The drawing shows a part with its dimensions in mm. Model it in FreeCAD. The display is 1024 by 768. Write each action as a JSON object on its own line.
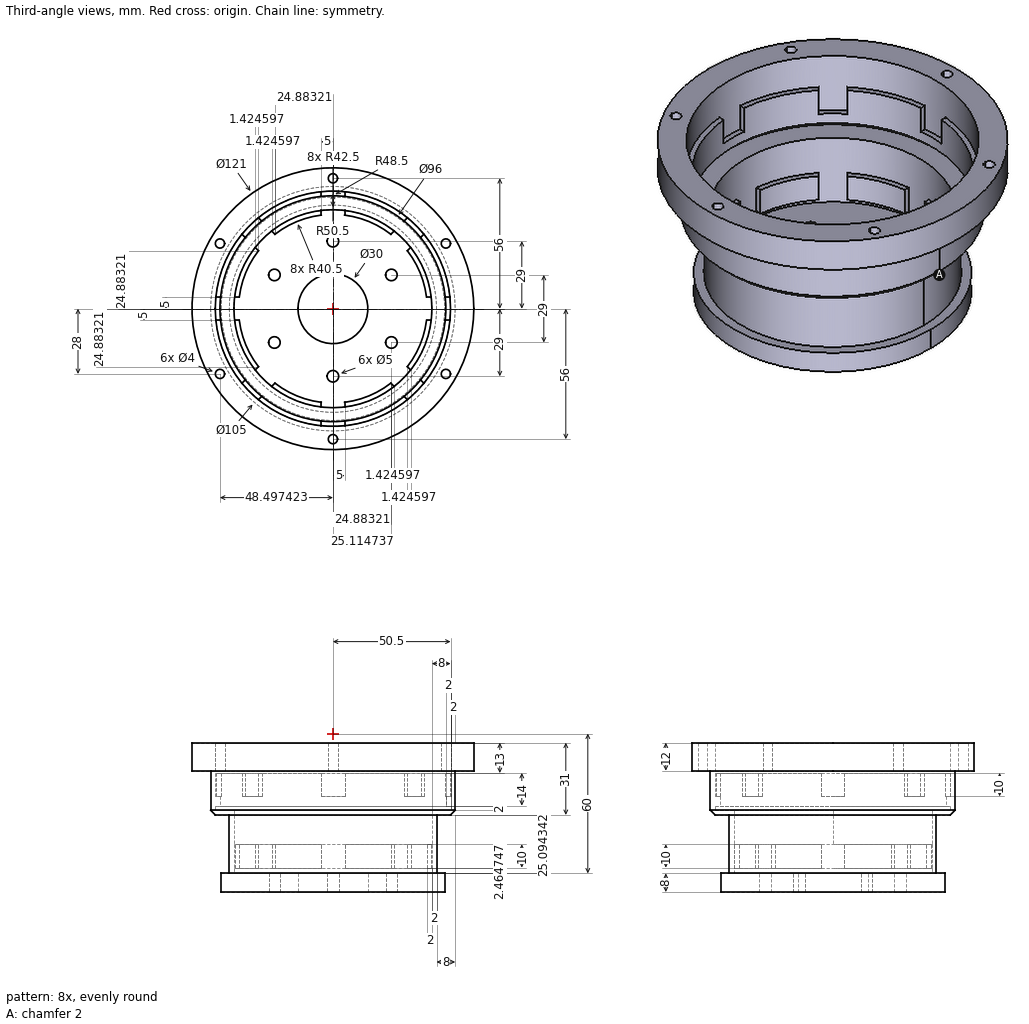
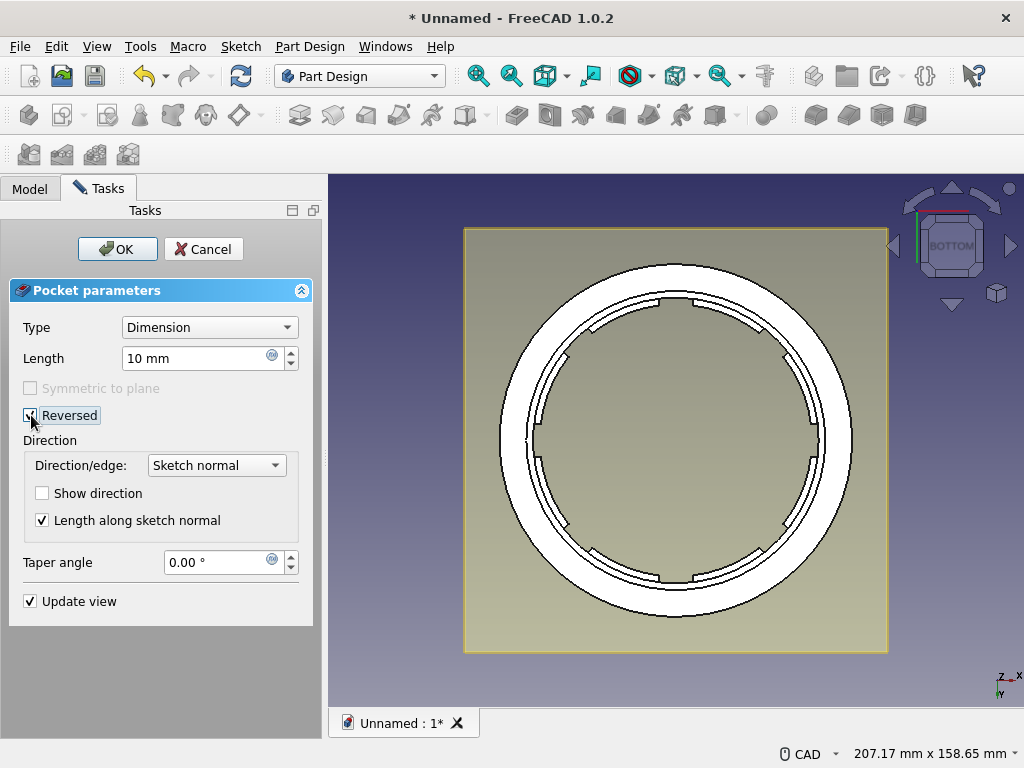
{"action": "left_click", "coordinate": [118, 249]}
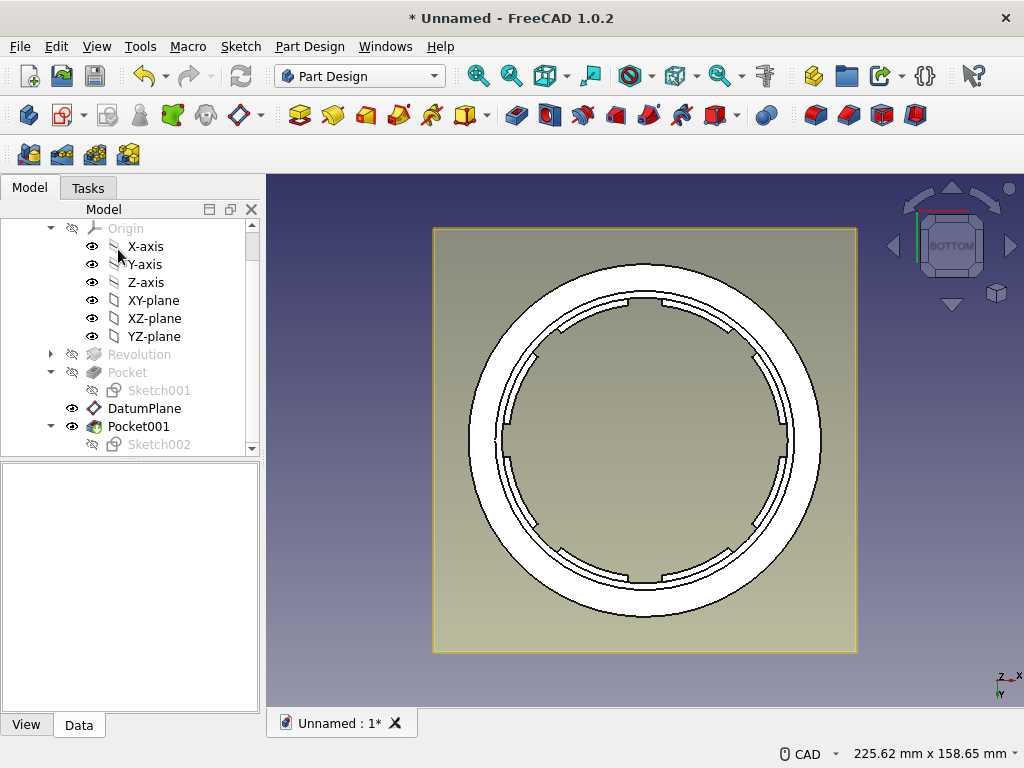
{"action": "left_click", "coordinate": [117, 408]}
{"action": "key", "text": "space"}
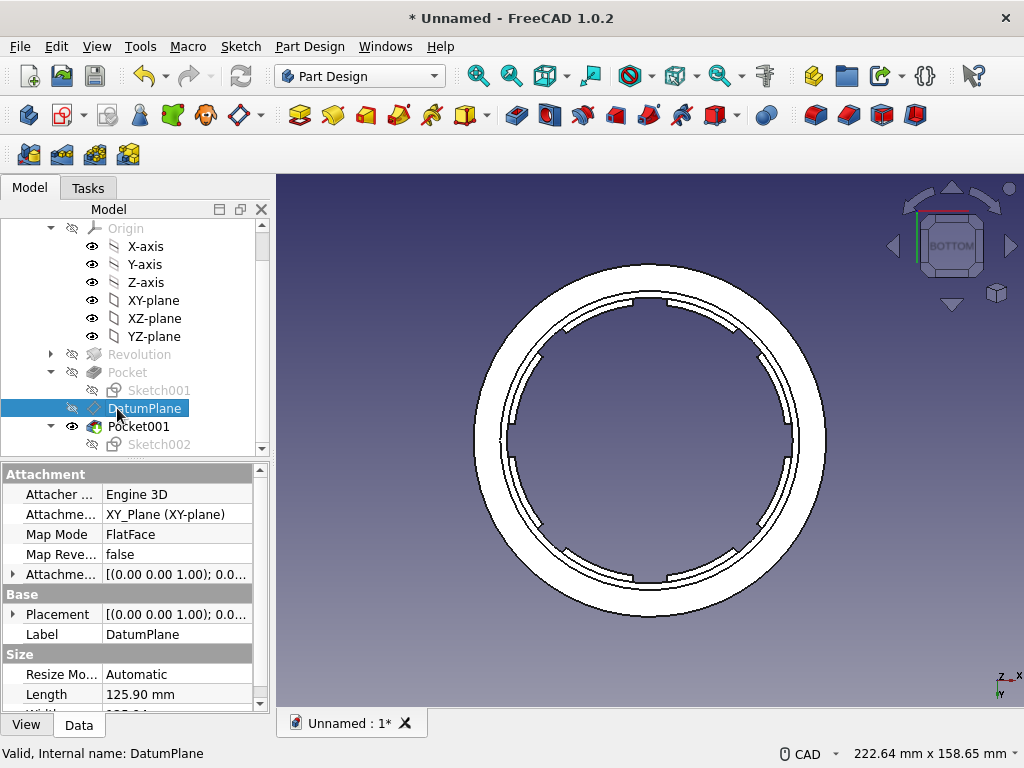
{"action": "left_click", "coordinate": [117, 426]}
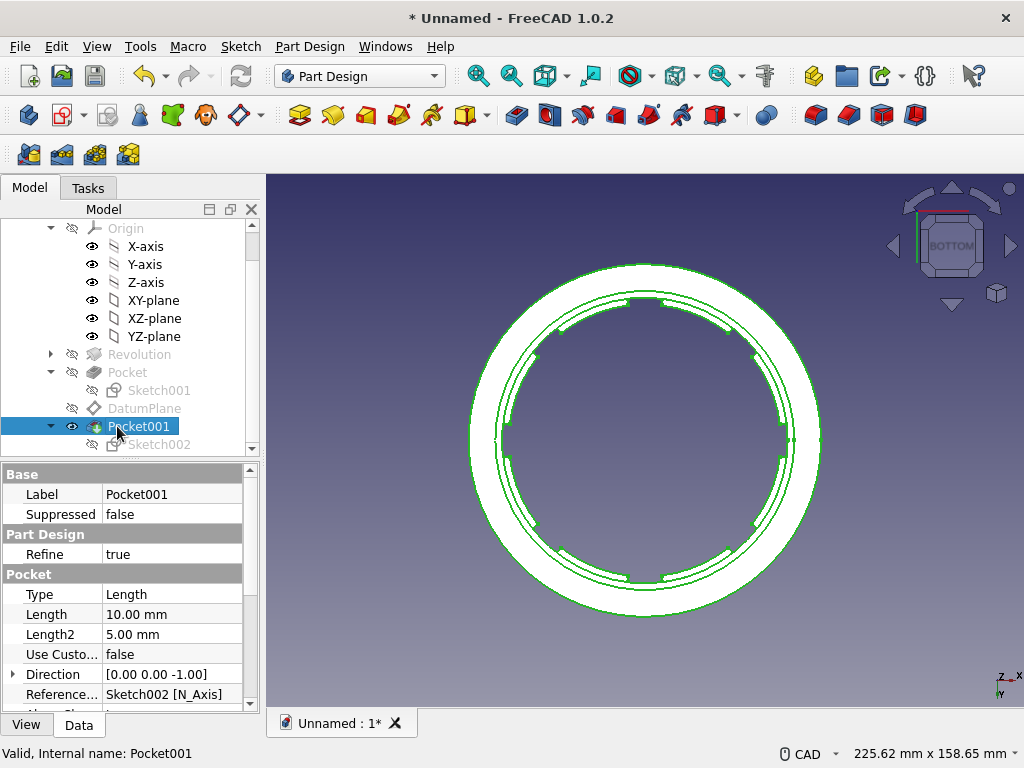
{"action": "left_click", "coordinate": [95, 154]}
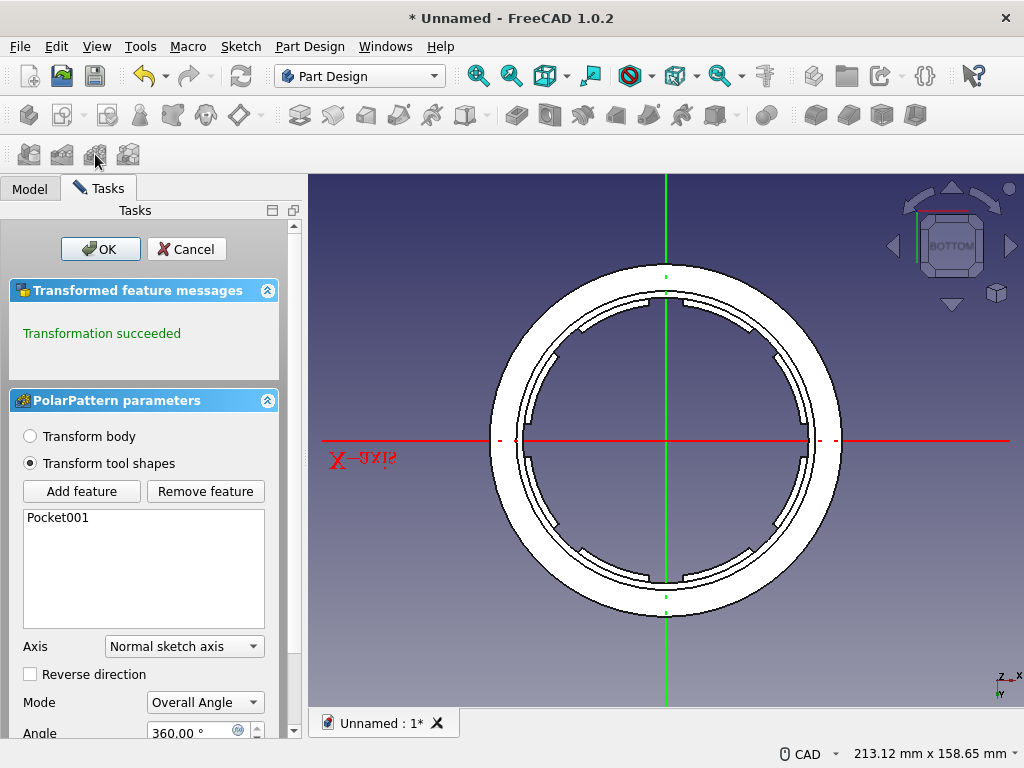
{"action": "left_click", "coordinate": [185, 646]}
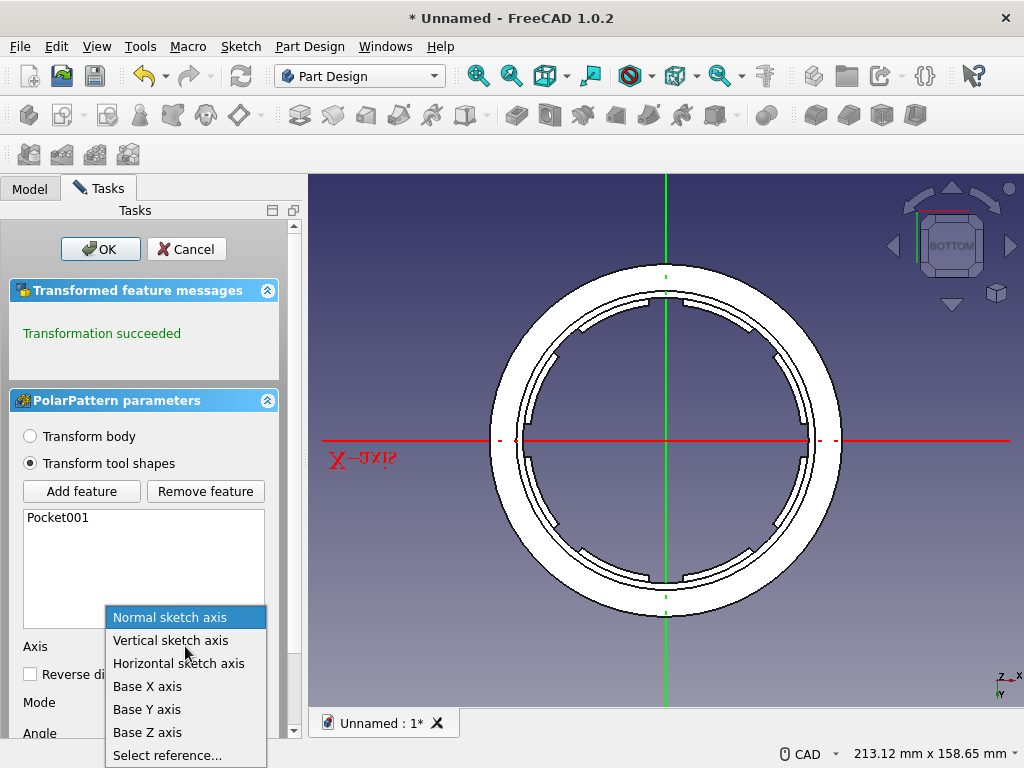
{"action": "left_click", "coordinate": [184, 732]}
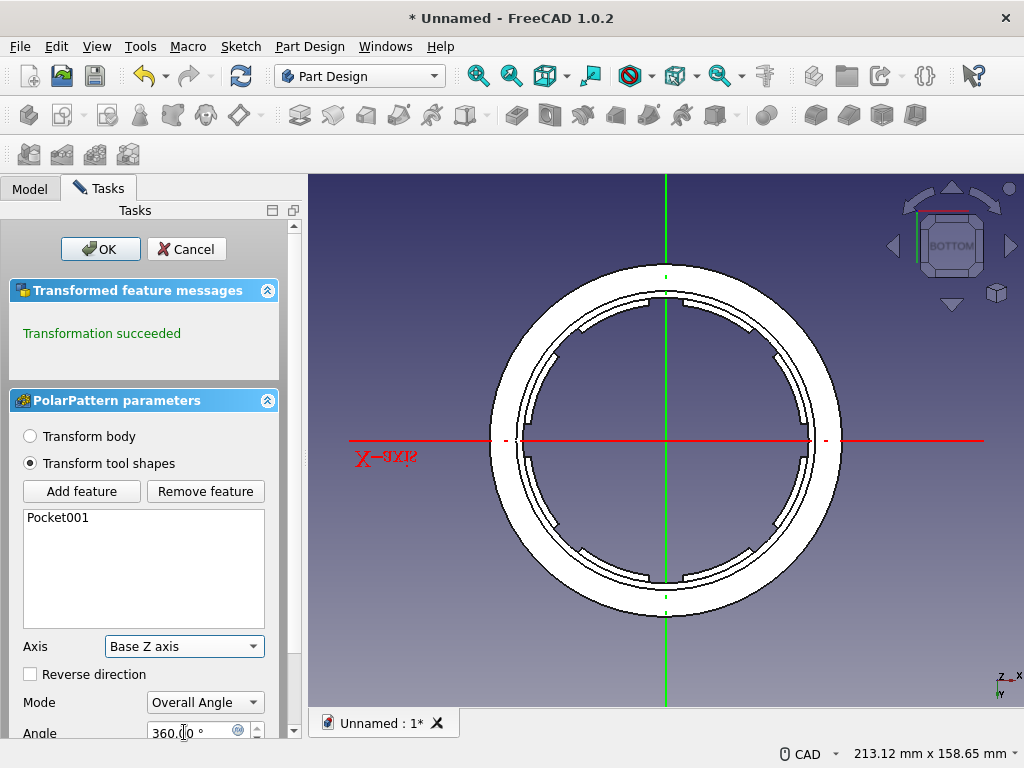
{"action": "scroll", "coordinate": [294, 479], "scroll_direction": "down", "scroll_amount": 2}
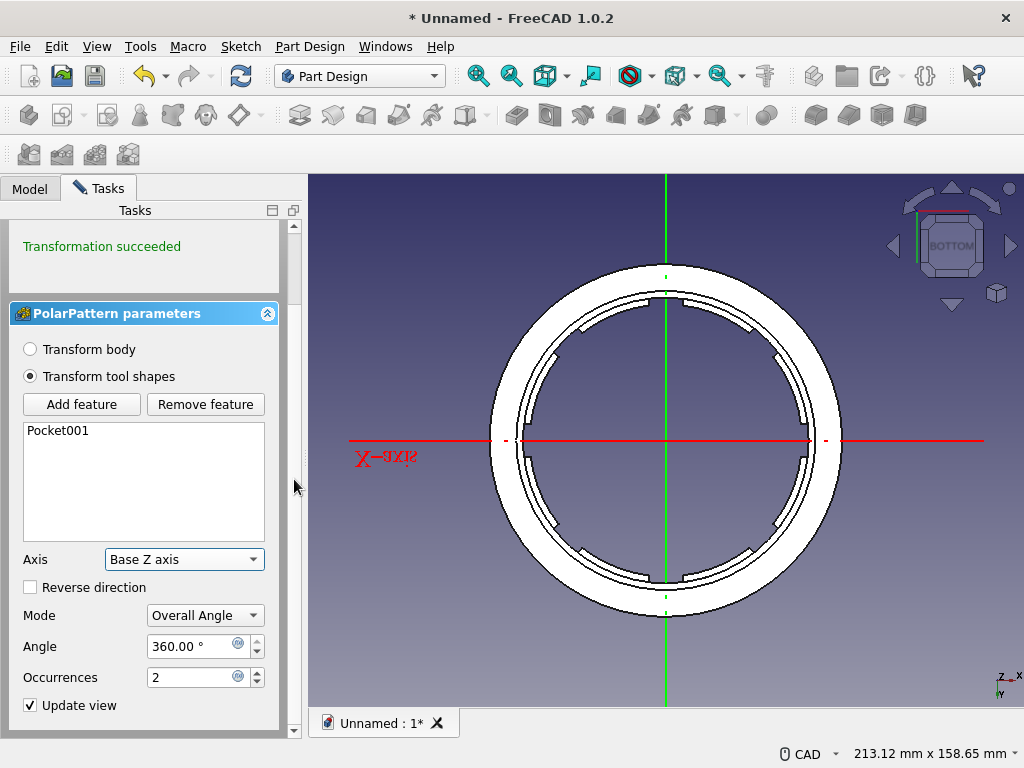
{"action": "triple_click", "coordinate": [199, 678]}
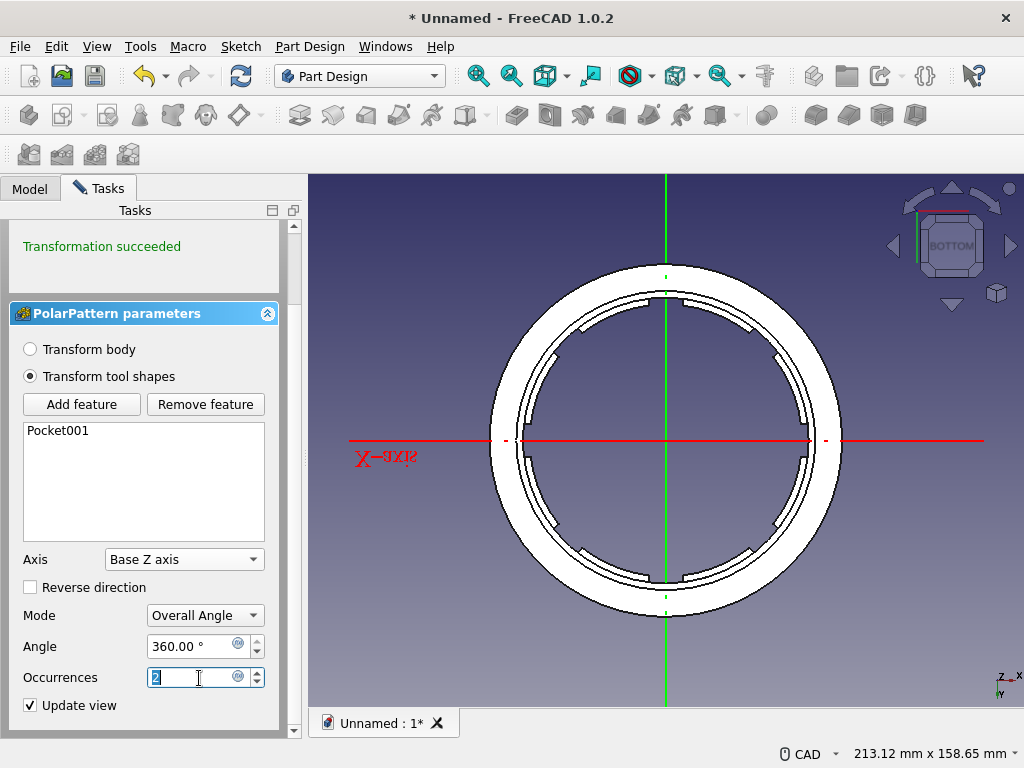
{"action": "type", "text": "8"}
{"action": "key", "text": "Tab"}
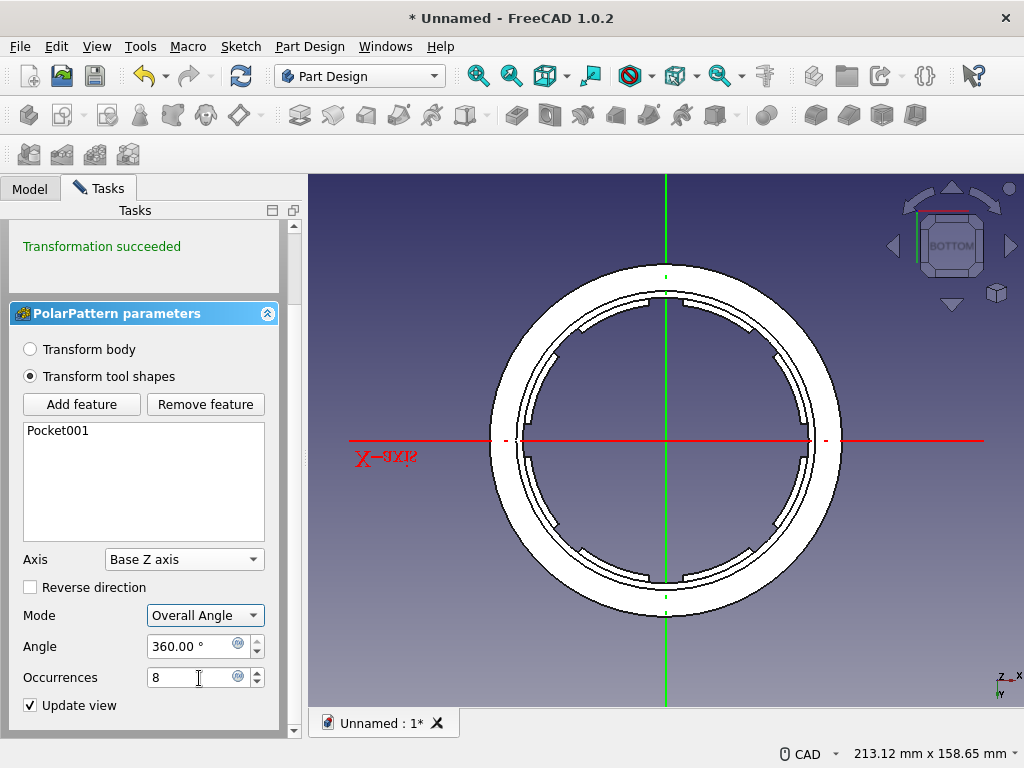
{"action": "scroll", "coordinate": [294, 479], "scroll_direction": "up", "scroll_amount": 3}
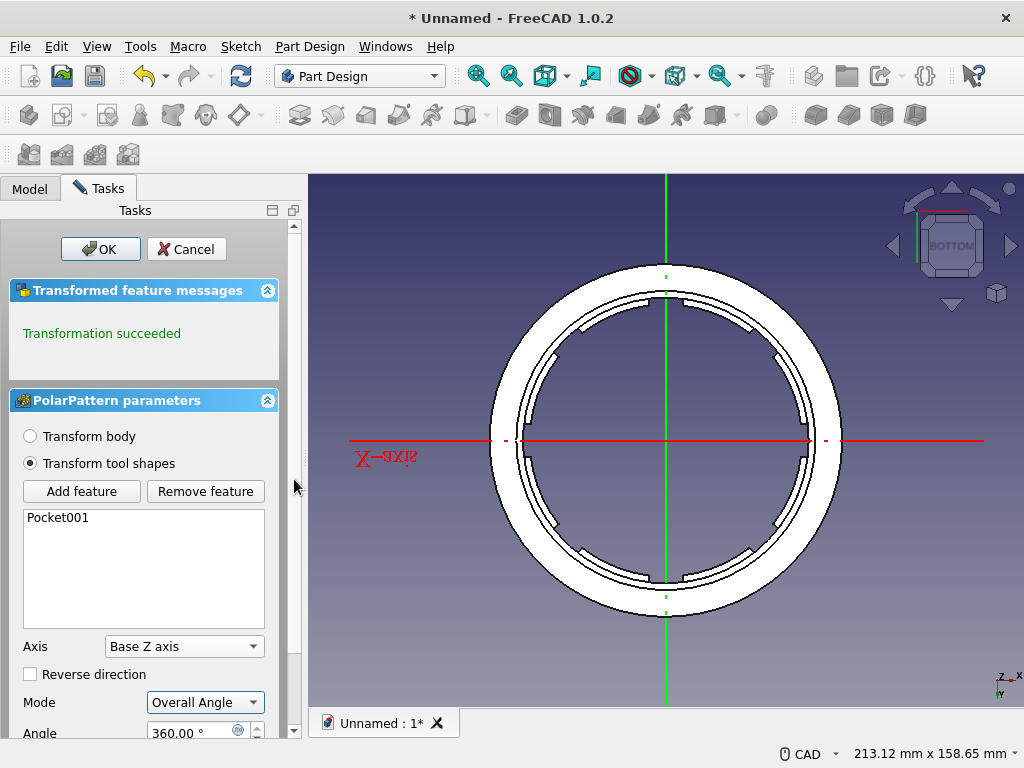
{"action": "left_click", "coordinate": [101, 249]}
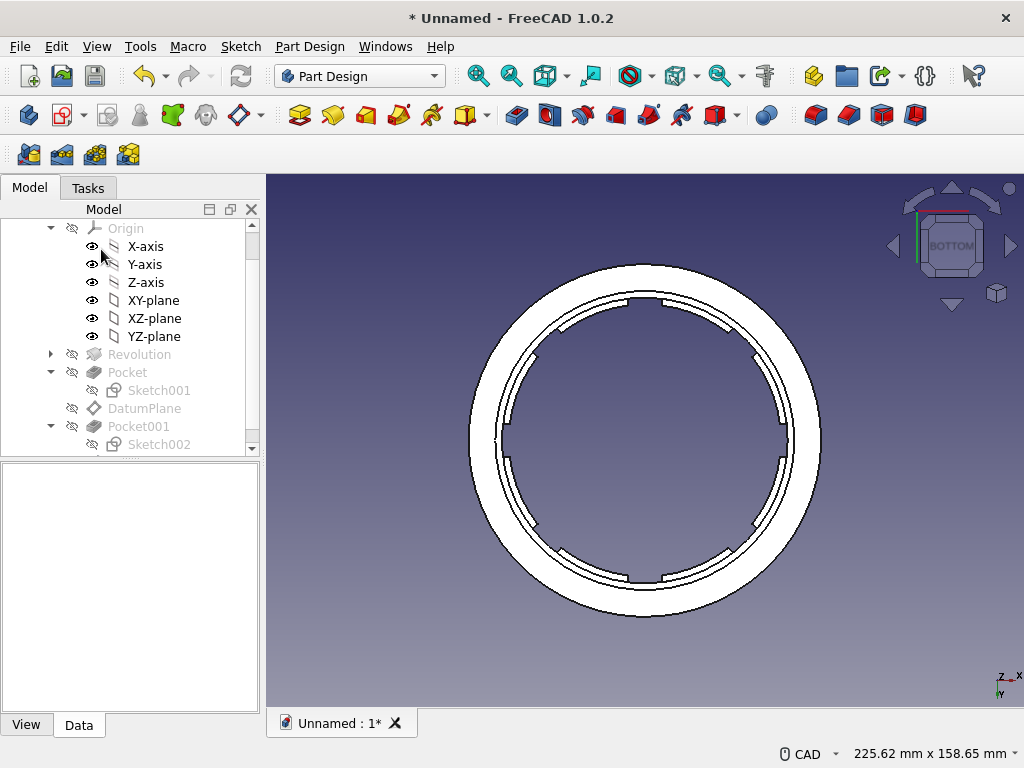
{"action": "left_click", "coordinate": [468, 439]}